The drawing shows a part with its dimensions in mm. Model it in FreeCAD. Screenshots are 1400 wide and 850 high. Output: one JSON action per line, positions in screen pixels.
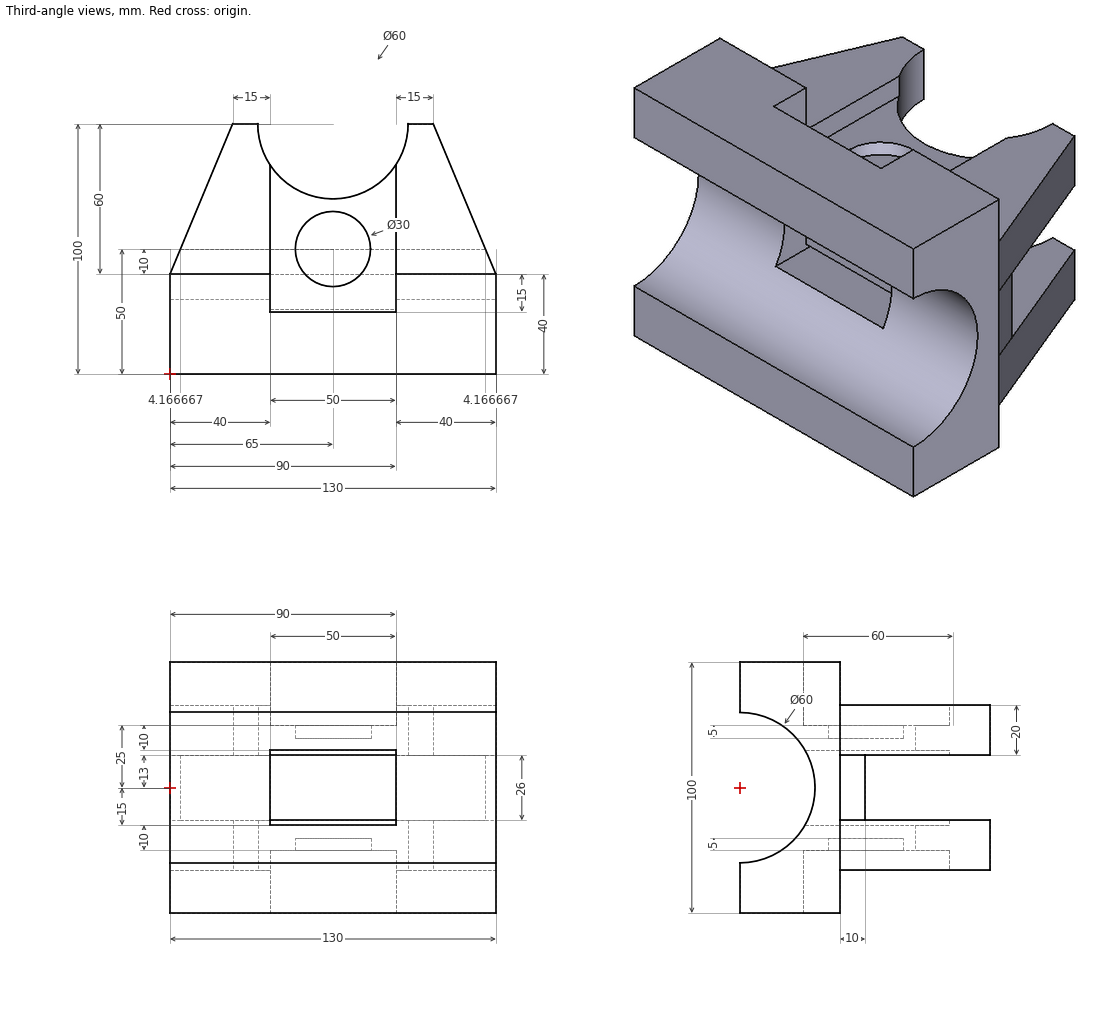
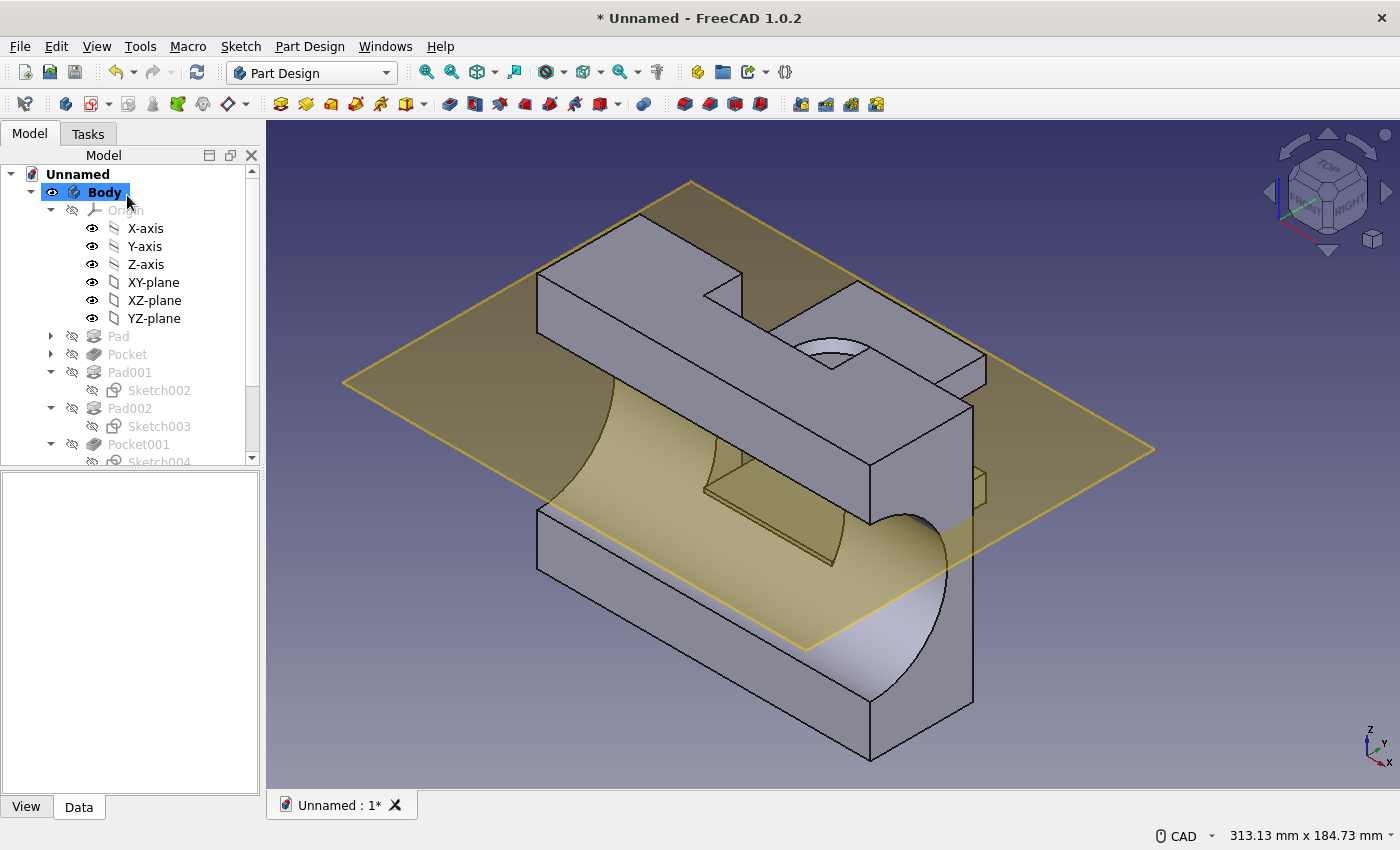
{"action": "scroll", "coordinate": [101, 314], "scroll_direction": "down", "scroll_amount": 3}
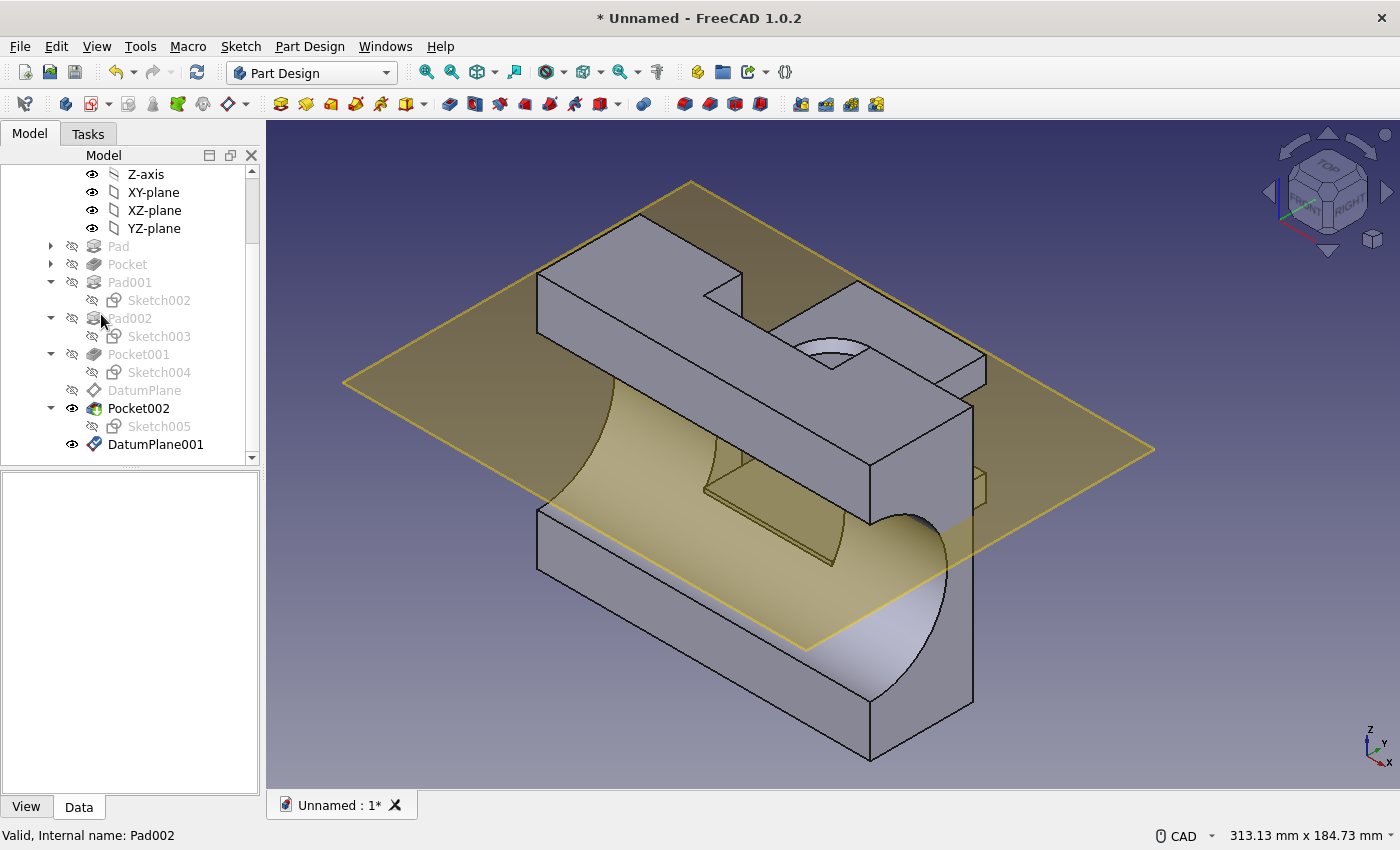
{"action": "left_click", "coordinate": [117, 444]}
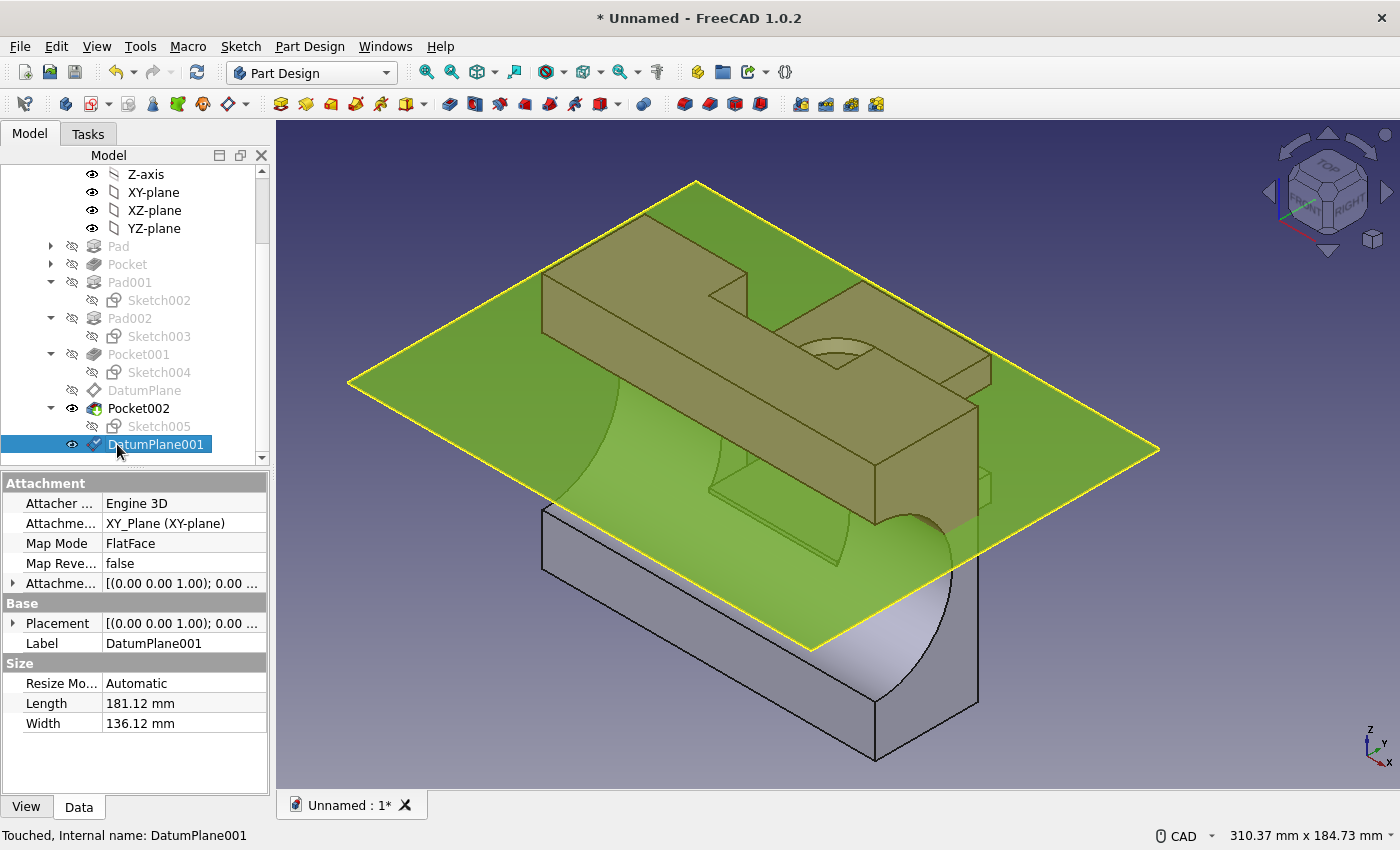
{"action": "left_click", "coordinate": [90, 104]}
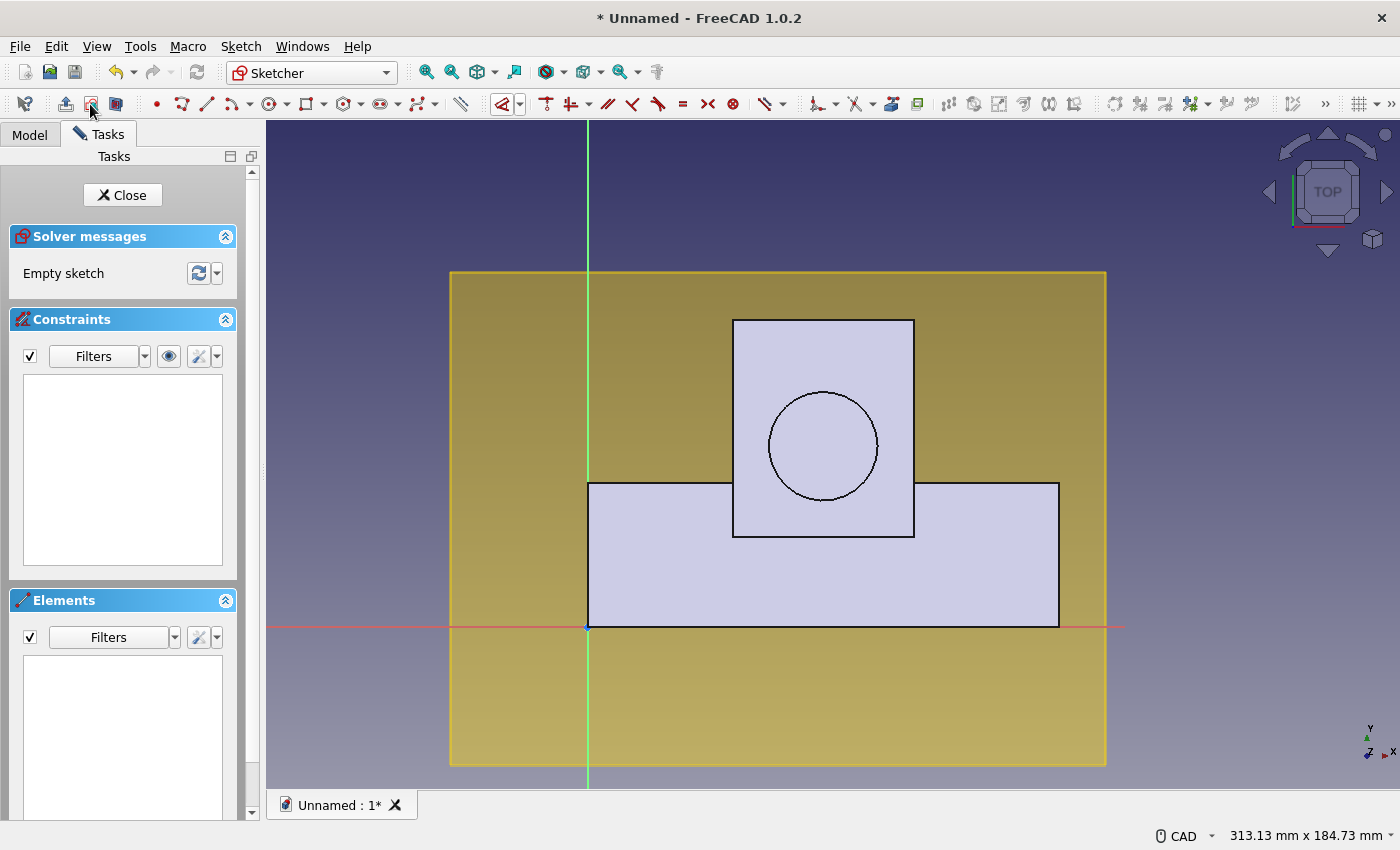
{"action": "left_click", "coordinate": [116, 104]}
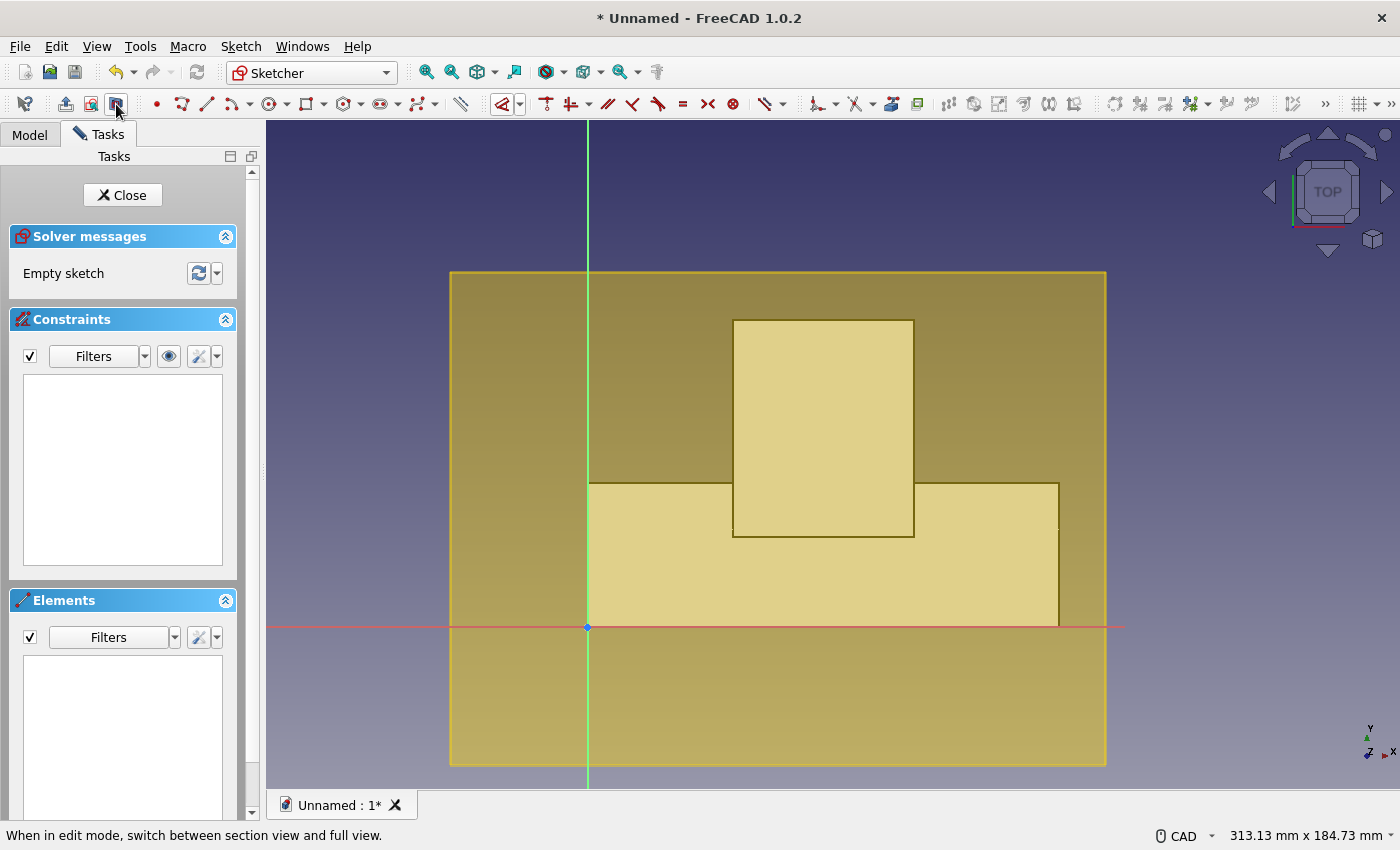
{"action": "left_click", "coordinate": [182, 104]}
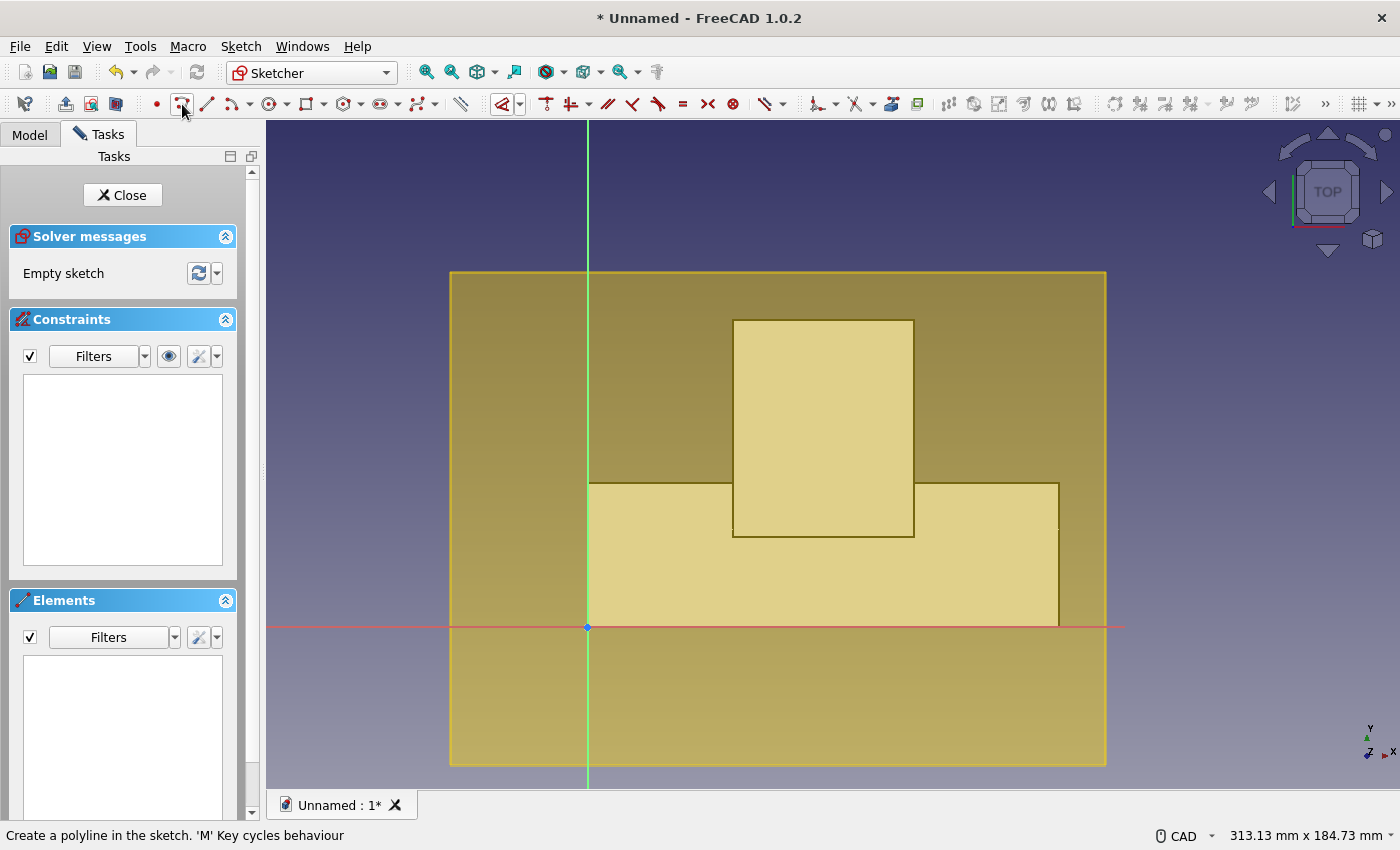
{"action": "left_click", "coordinate": [588, 483]}
{"action": "left_click", "coordinate": [733, 483]}
{"action": "left_click", "coordinate": [733, 265]}
{"action": "left_click", "coordinate": [678, 265]}
{"action": "left_click", "coordinate": [588, 484]}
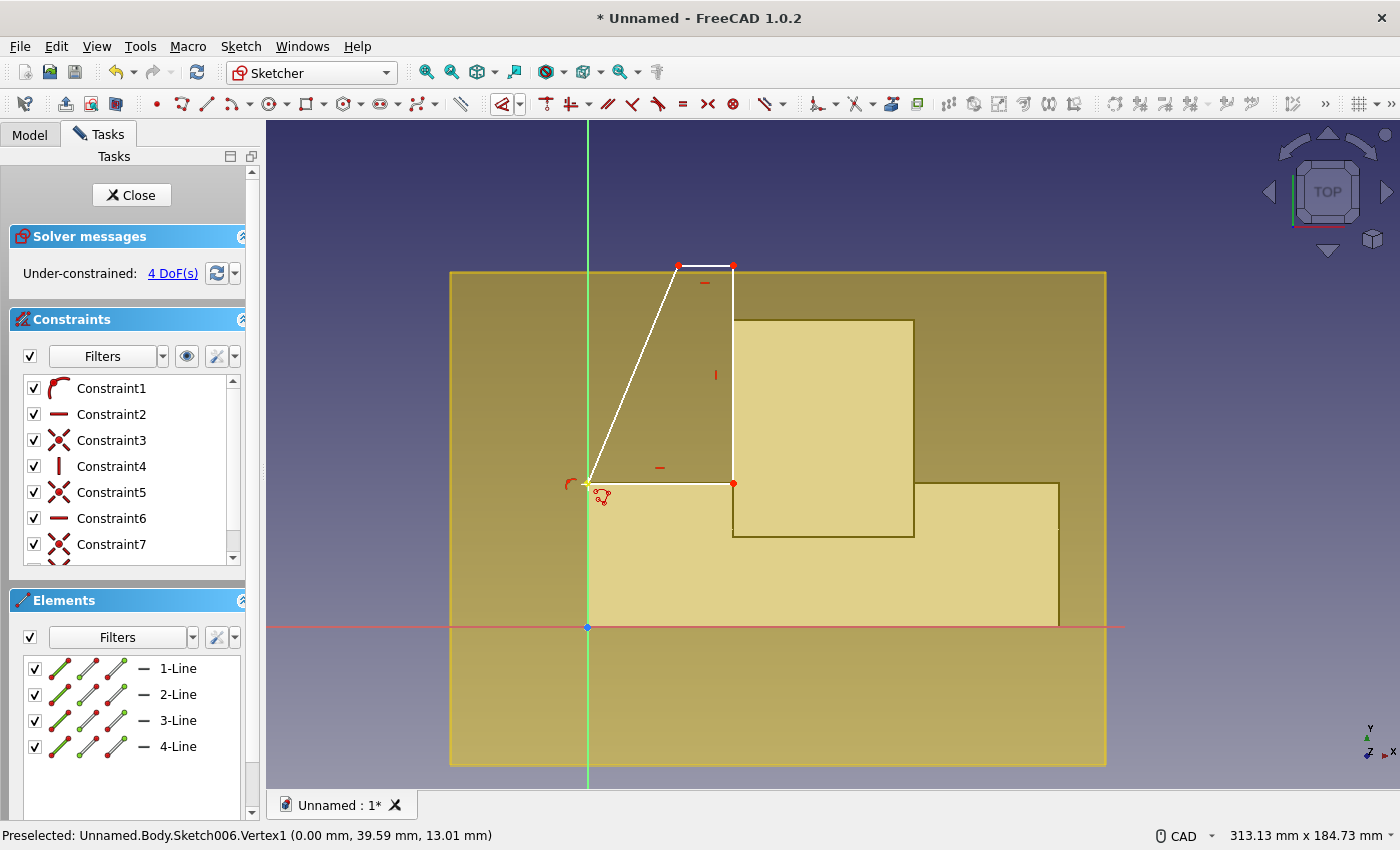
{"action": "left_click", "coordinate": [914, 483]}
{"action": "left_click", "coordinate": [1059, 483]}
{"action": "left_click", "coordinate": [968, 265]}
{"action": "left_click", "coordinate": [914, 265]}
{"action": "left_click", "coordinate": [914, 484]}
{"action": "key", "text": "Escape"}
{"action": "key", "text": "Escape"}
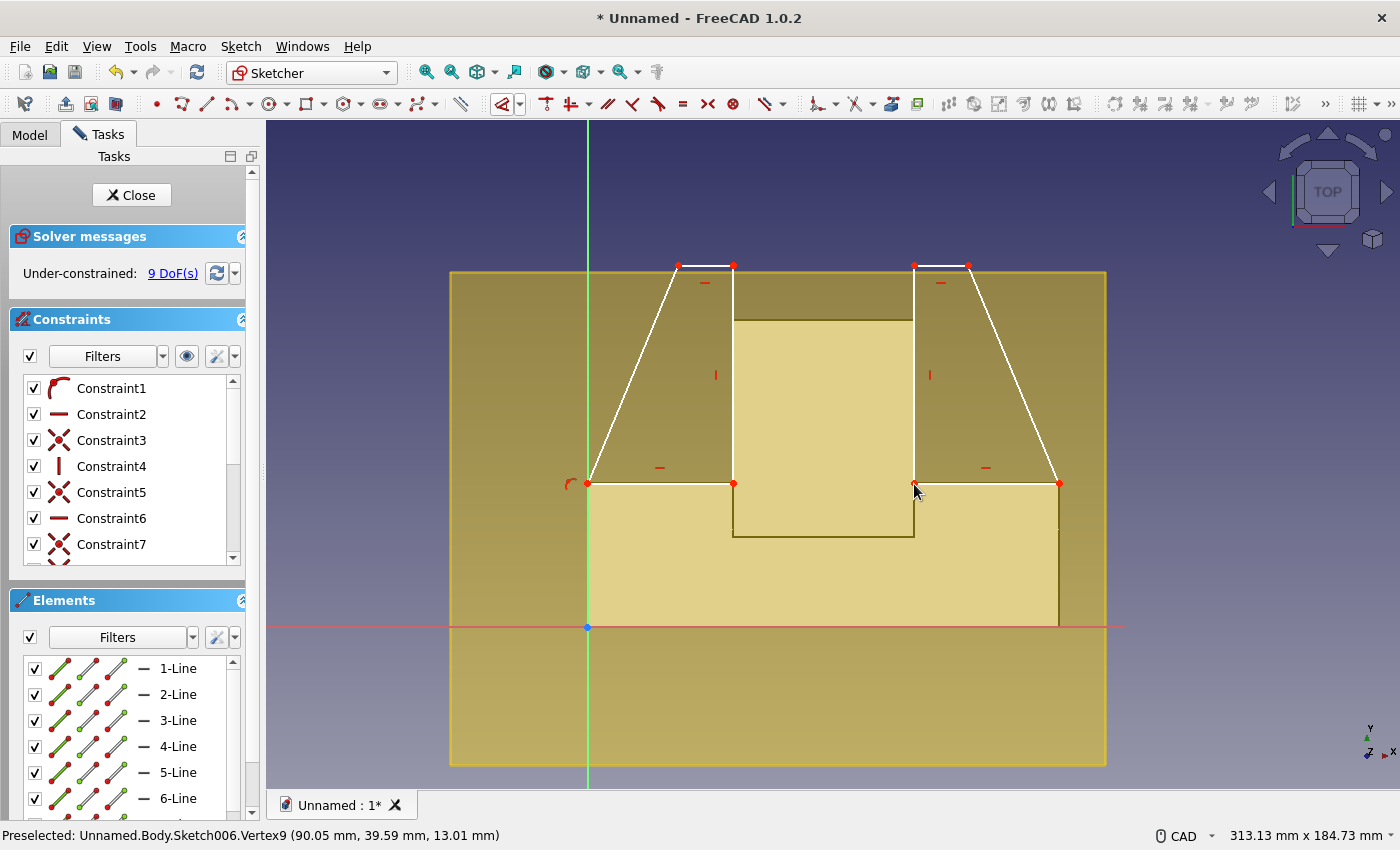
{"action": "left_click", "coordinate": [631, 484]}